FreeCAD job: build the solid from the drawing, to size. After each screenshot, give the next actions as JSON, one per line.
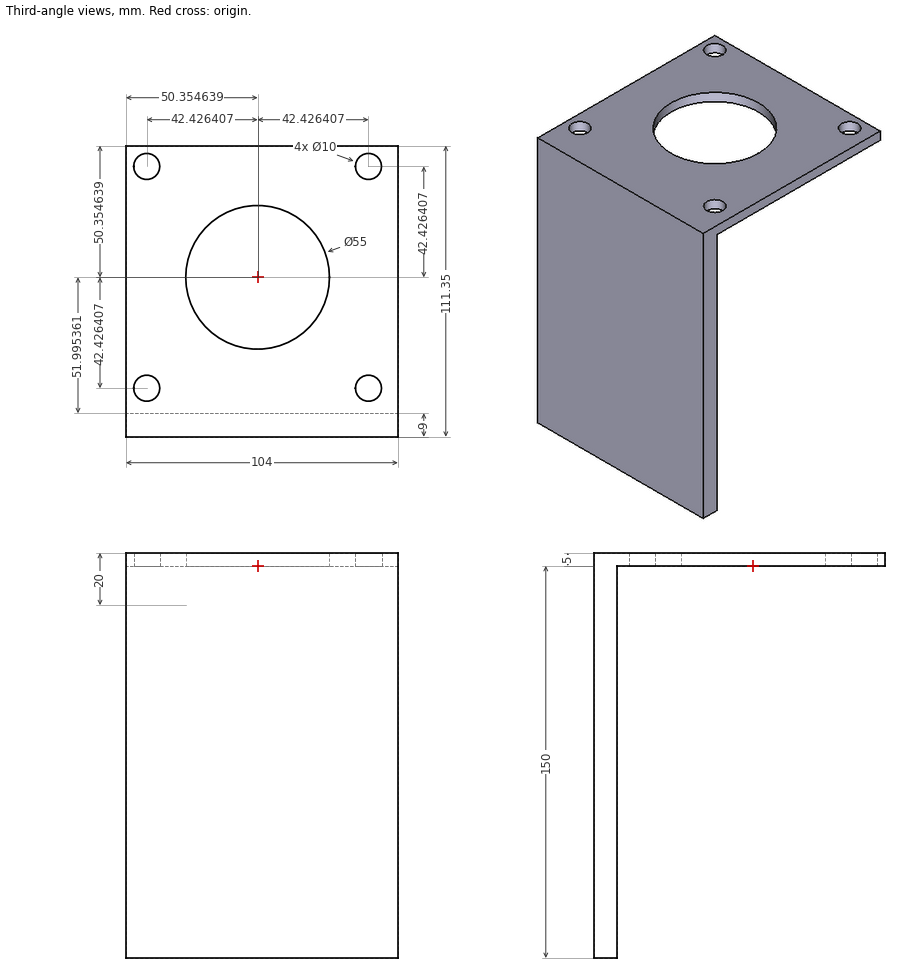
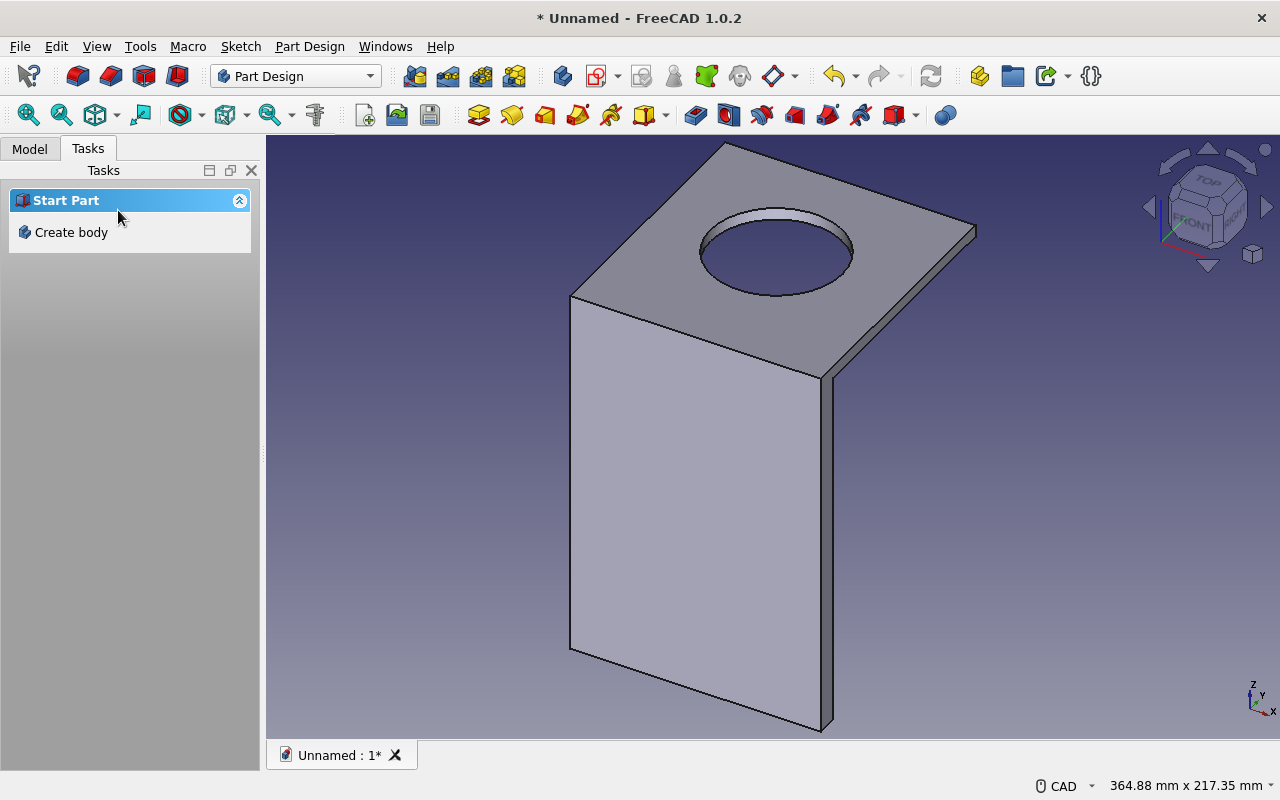
{"action": "left_click", "coordinate": [596, 76]}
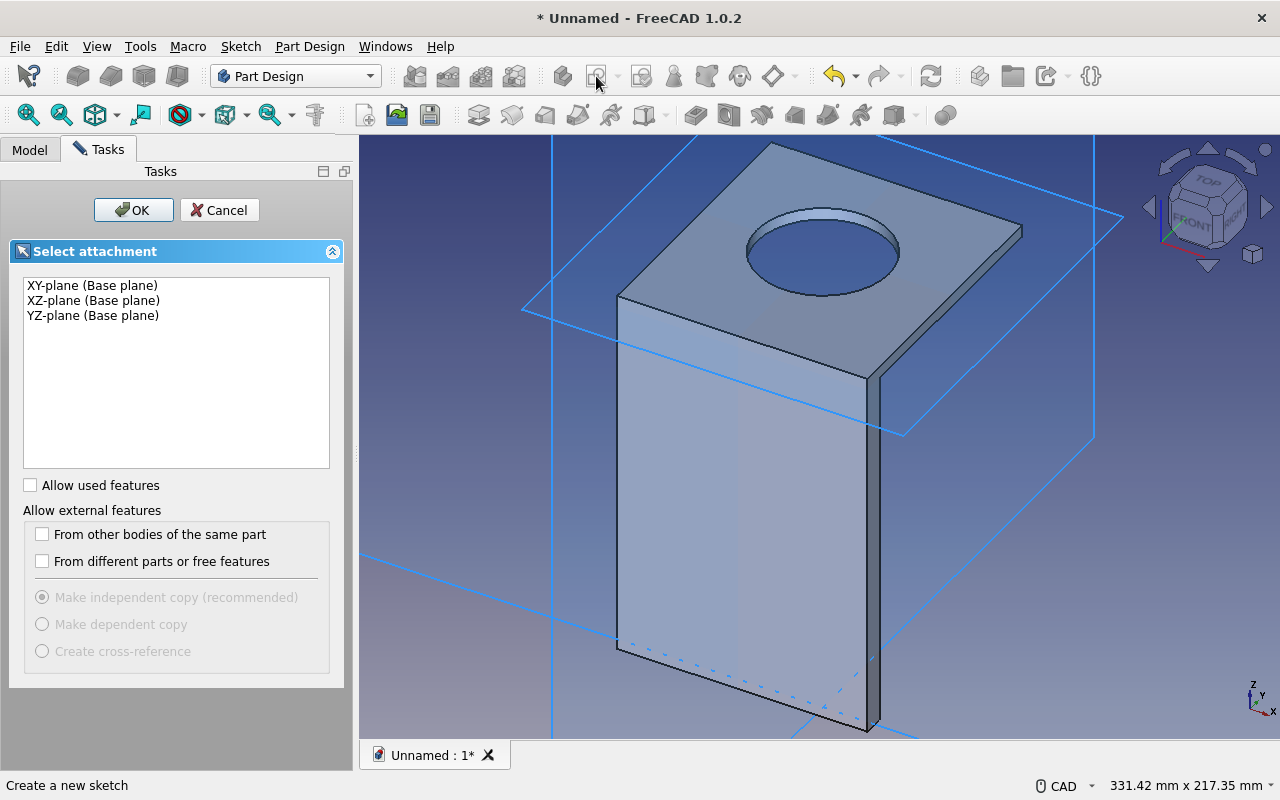
{"action": "left_click", "coordinate": [84, 286]}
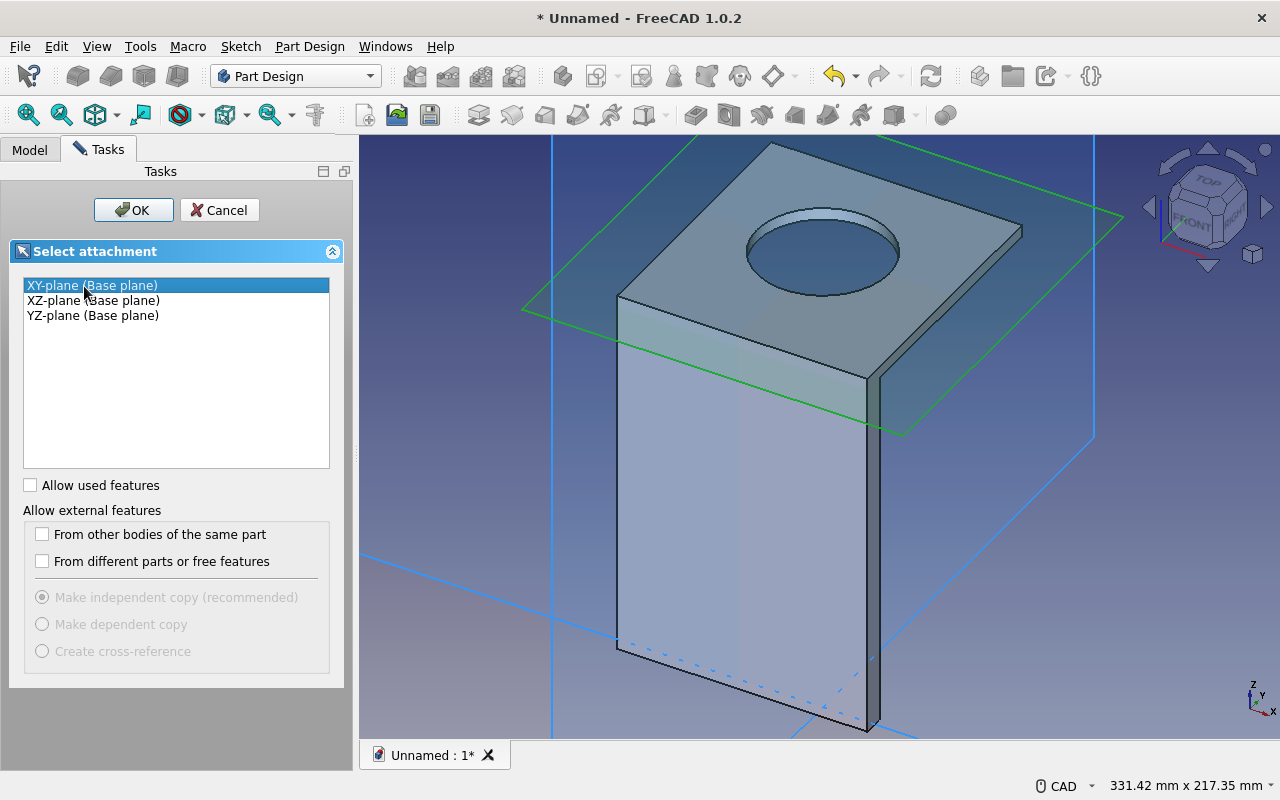
{"action": "left_click", "coordinate": [134, 210]}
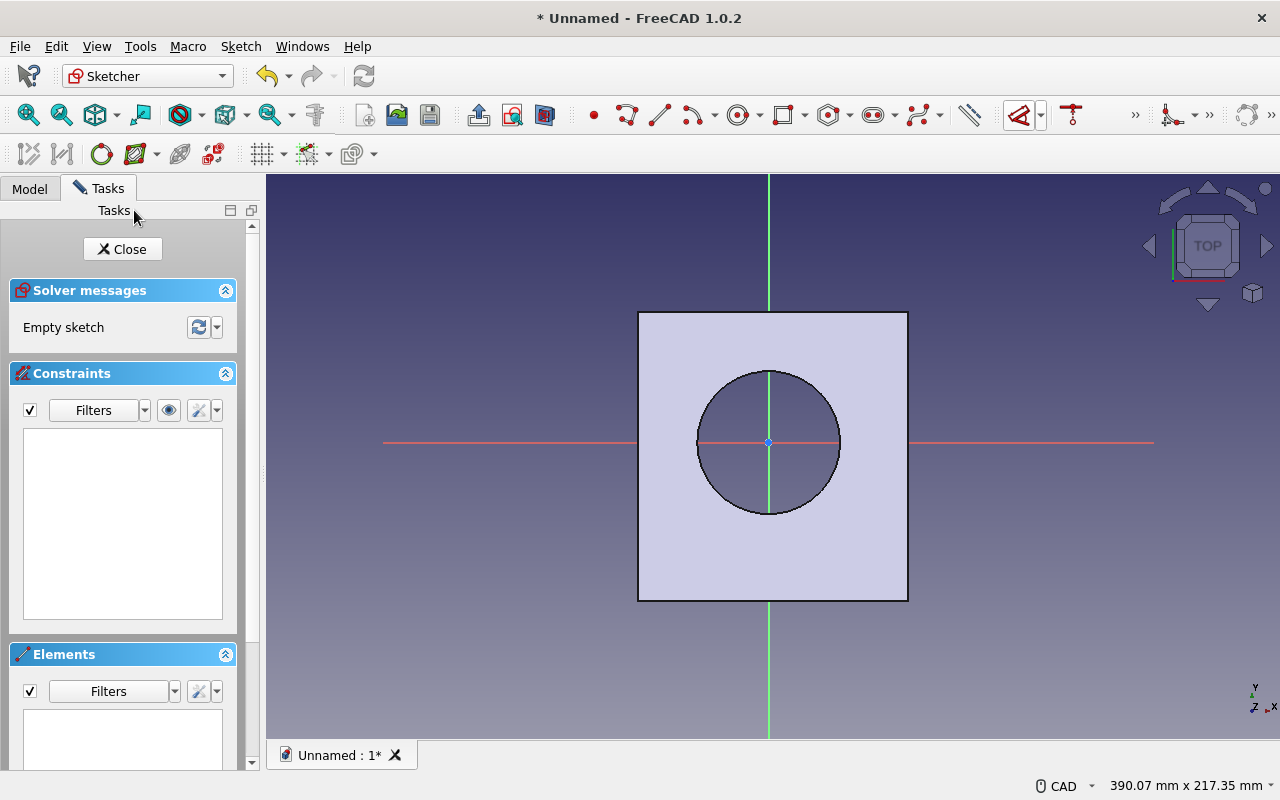
{"action": "left_click", "coordinate": [545, 116]}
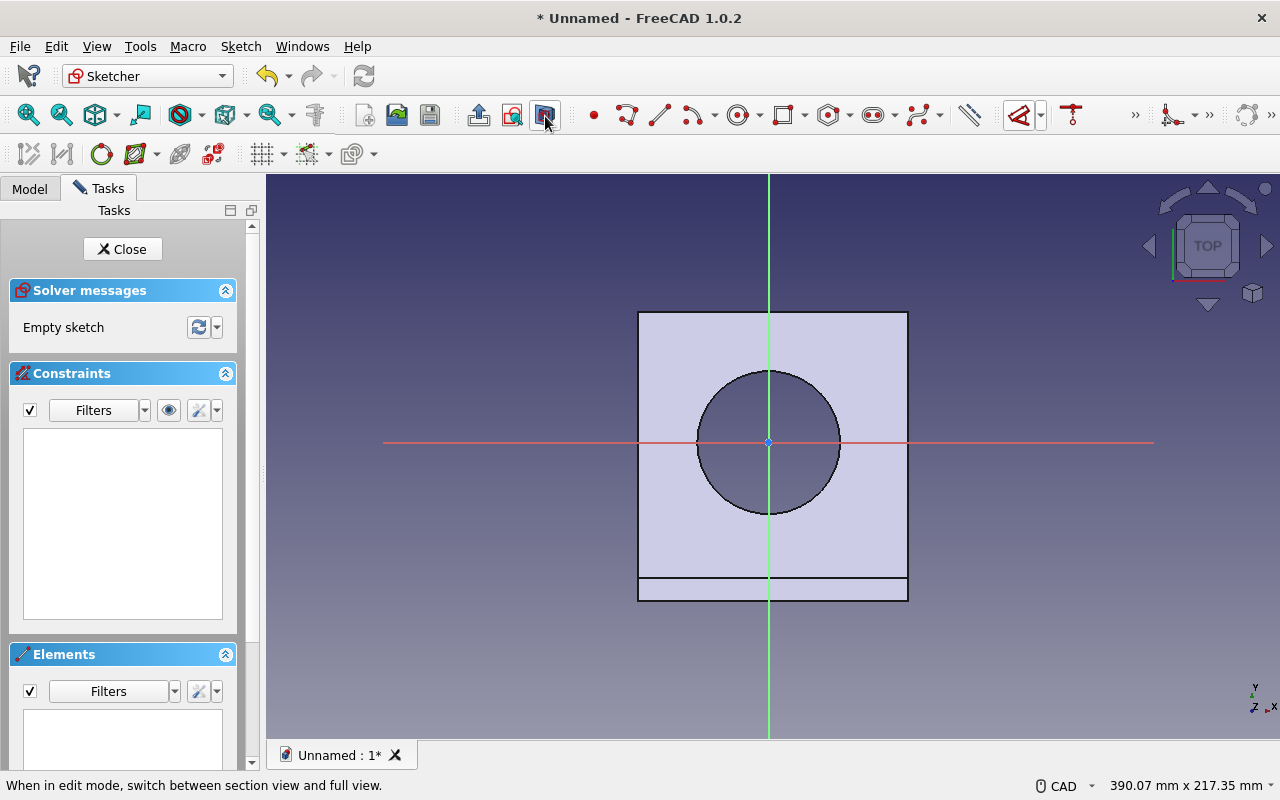
{"action": "scroll", "coordinate": [899, 415], "scroll_direction": "up", "scroll_amount": 2}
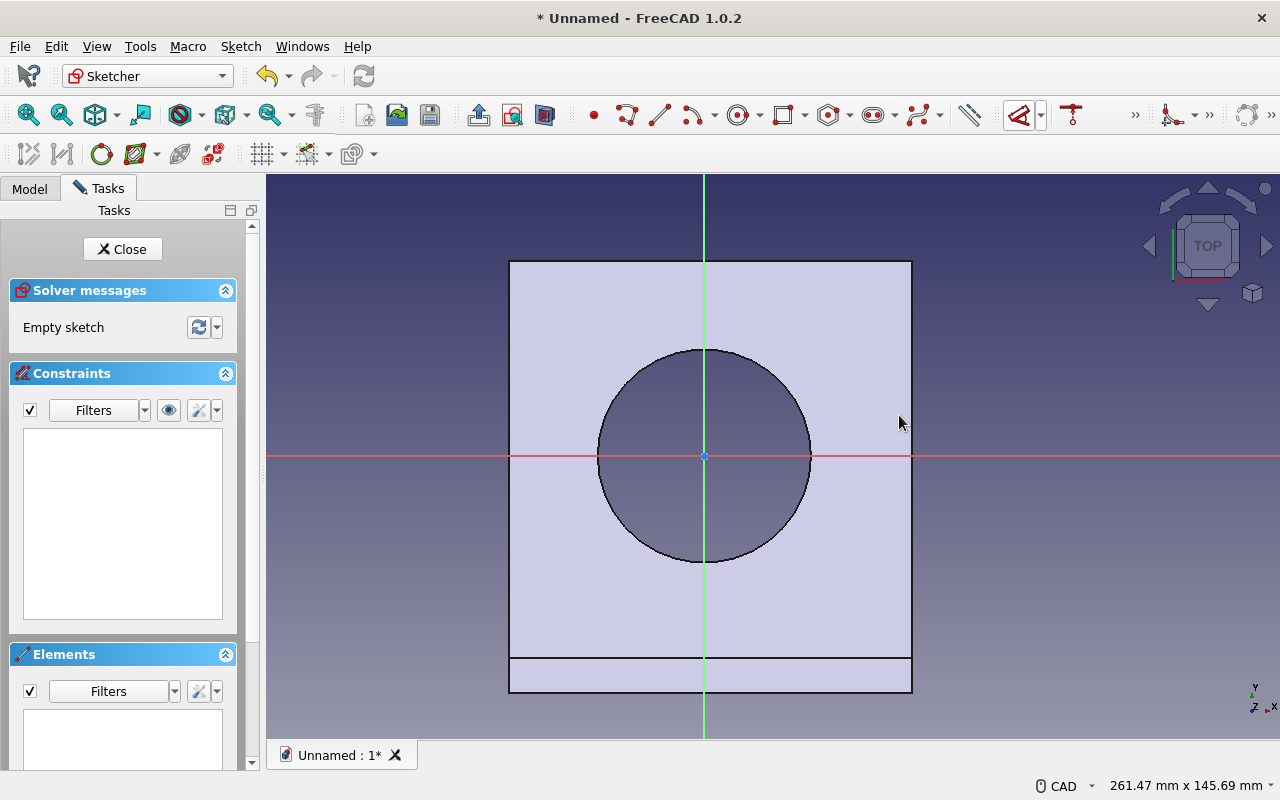
{"action": "left_click", "coordinate": [738, 116]}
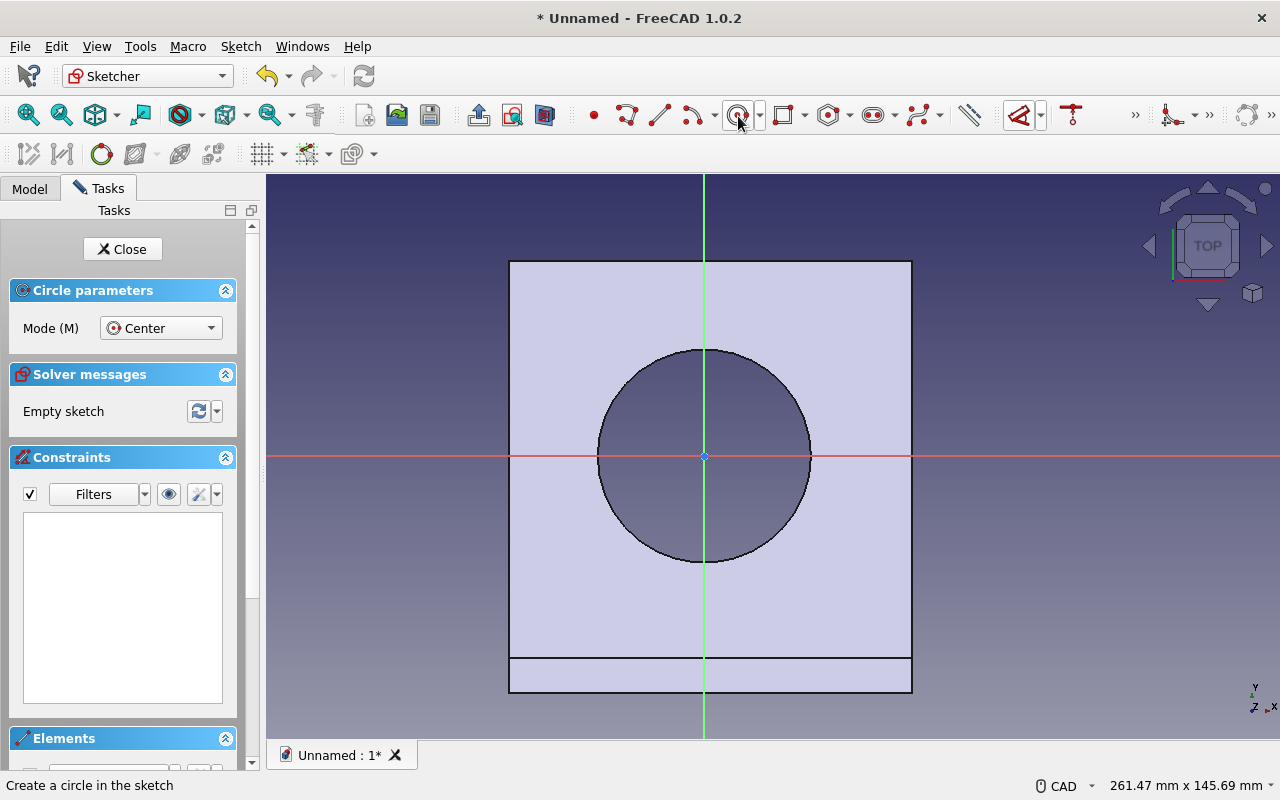
{"action": "left_click", "coordinate": [869, 292]}
{"action": "mouse_move", "coordinate": [883, 278]}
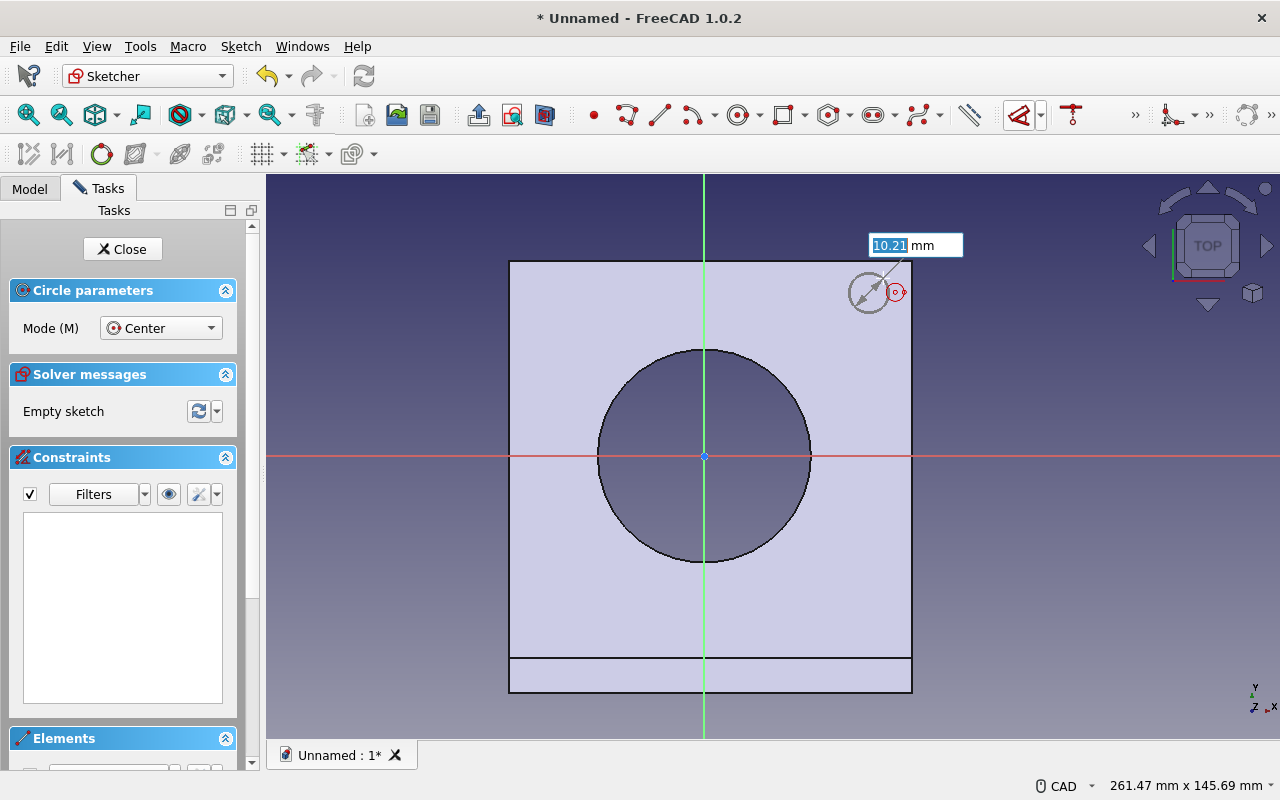
{"action": "type", "text": "10"}
{"action": "key", "text": "Return"}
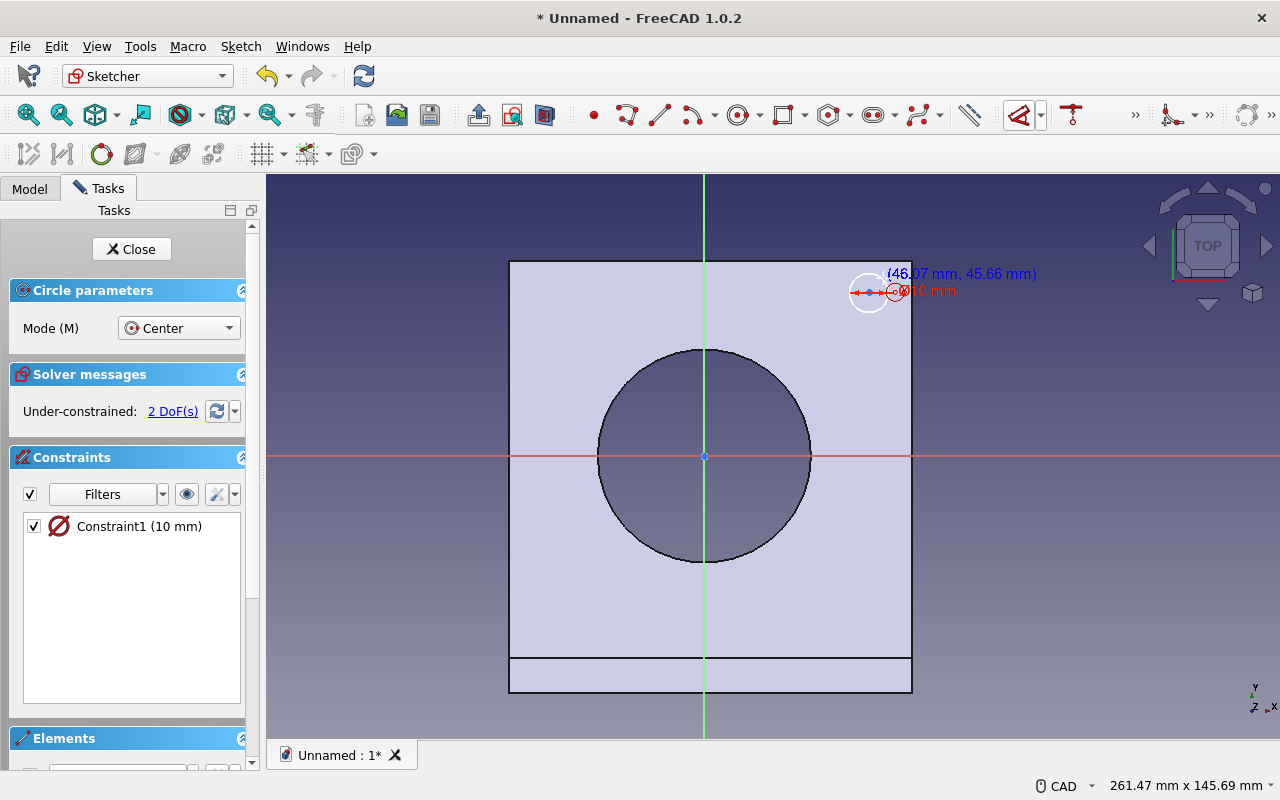
{"action": "left_click", "coordinate": [540, 292]}
{"action": "mouse_move", "coordinate": [554, 278]}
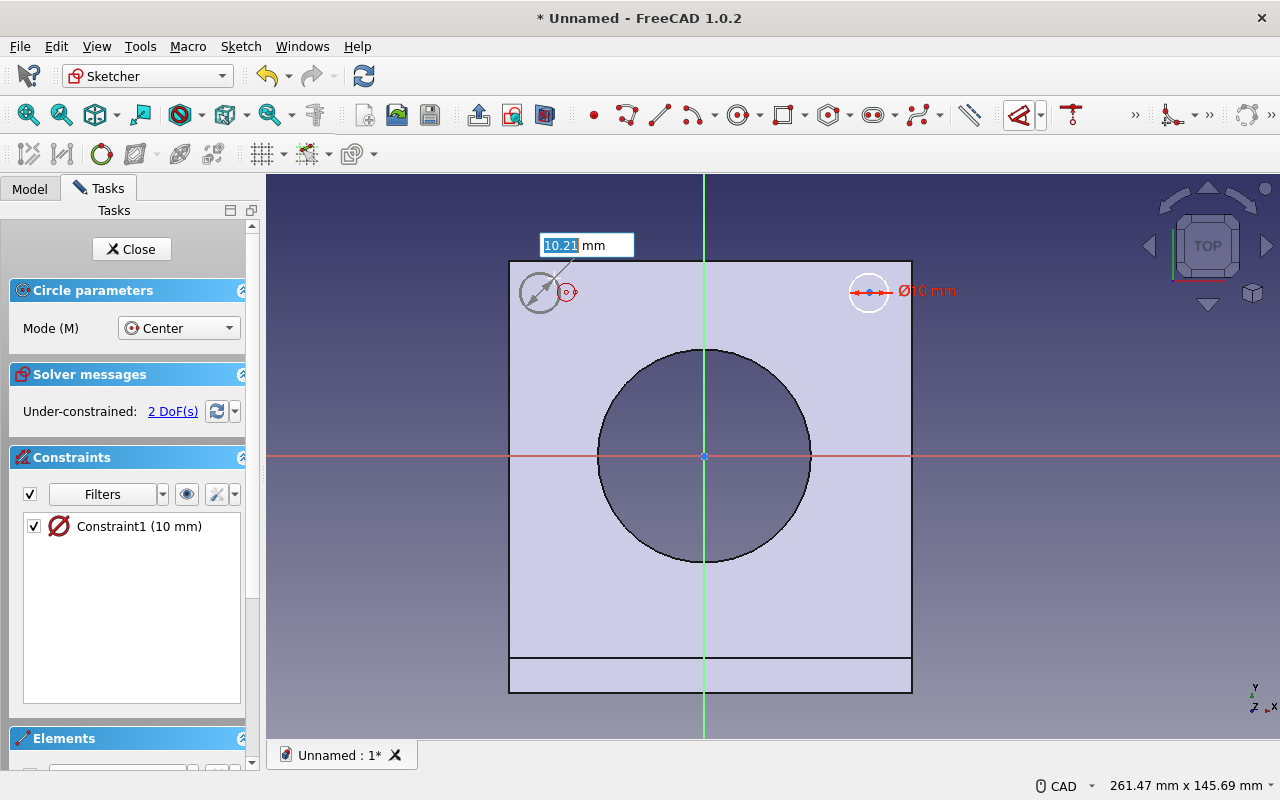
{"action": "type", "text": "10"}
{"action": "key", "text": "Return"}